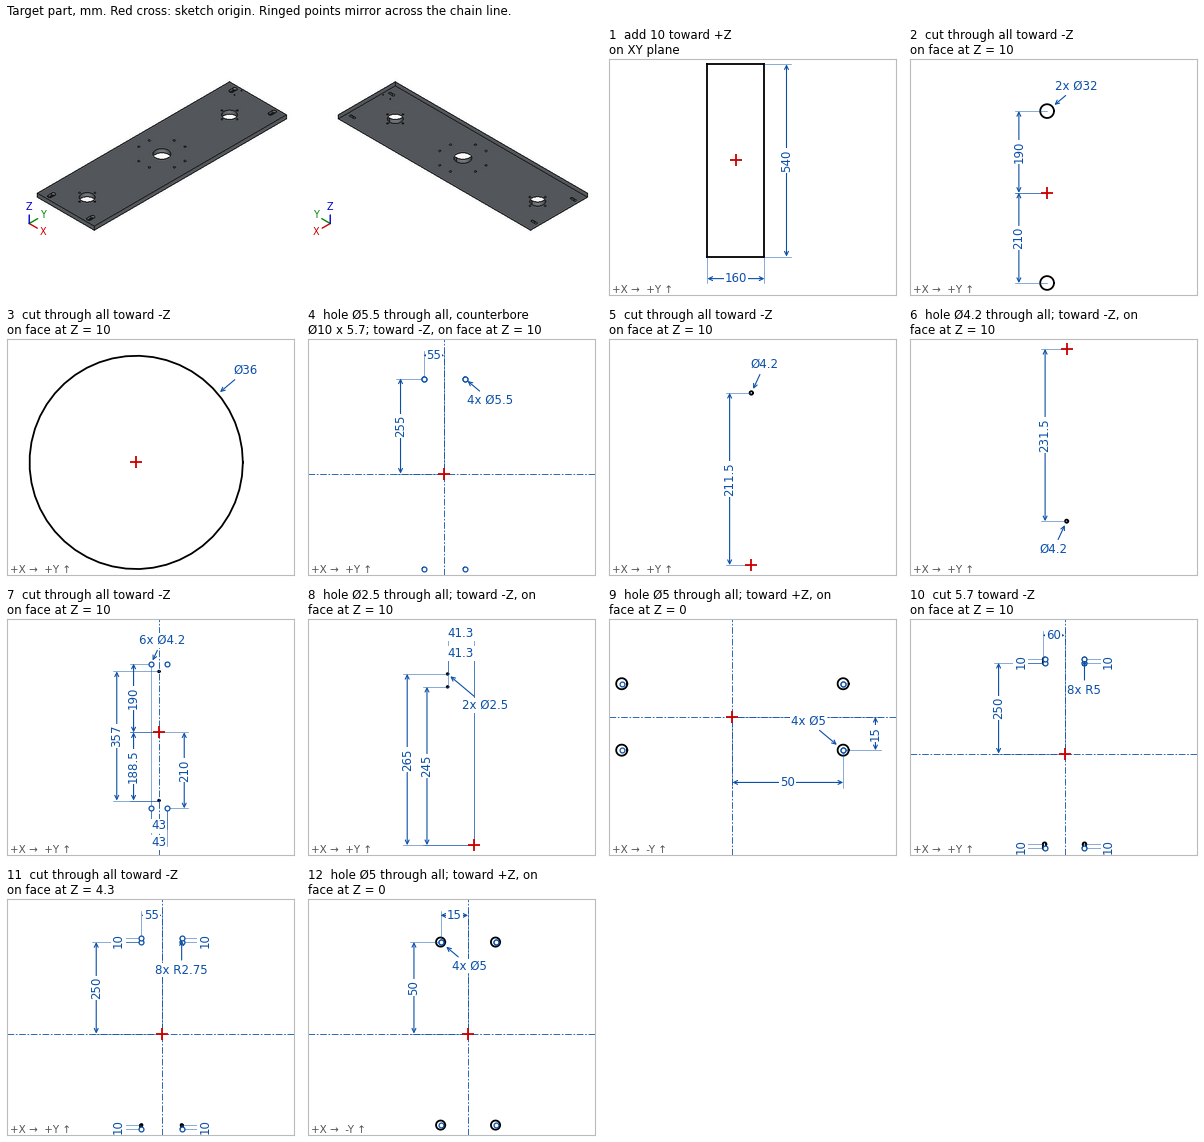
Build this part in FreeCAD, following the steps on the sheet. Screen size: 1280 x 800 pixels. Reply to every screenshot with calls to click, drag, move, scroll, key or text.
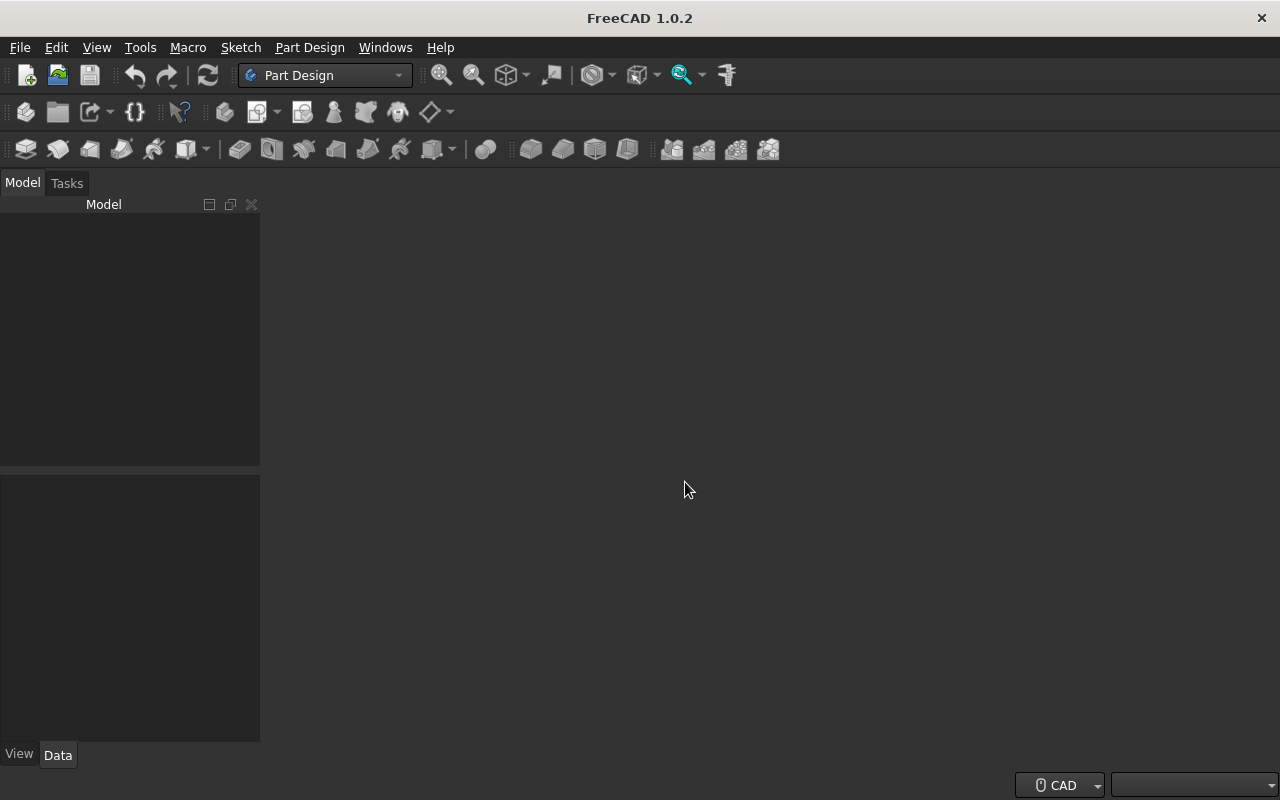
key(ctrl+n)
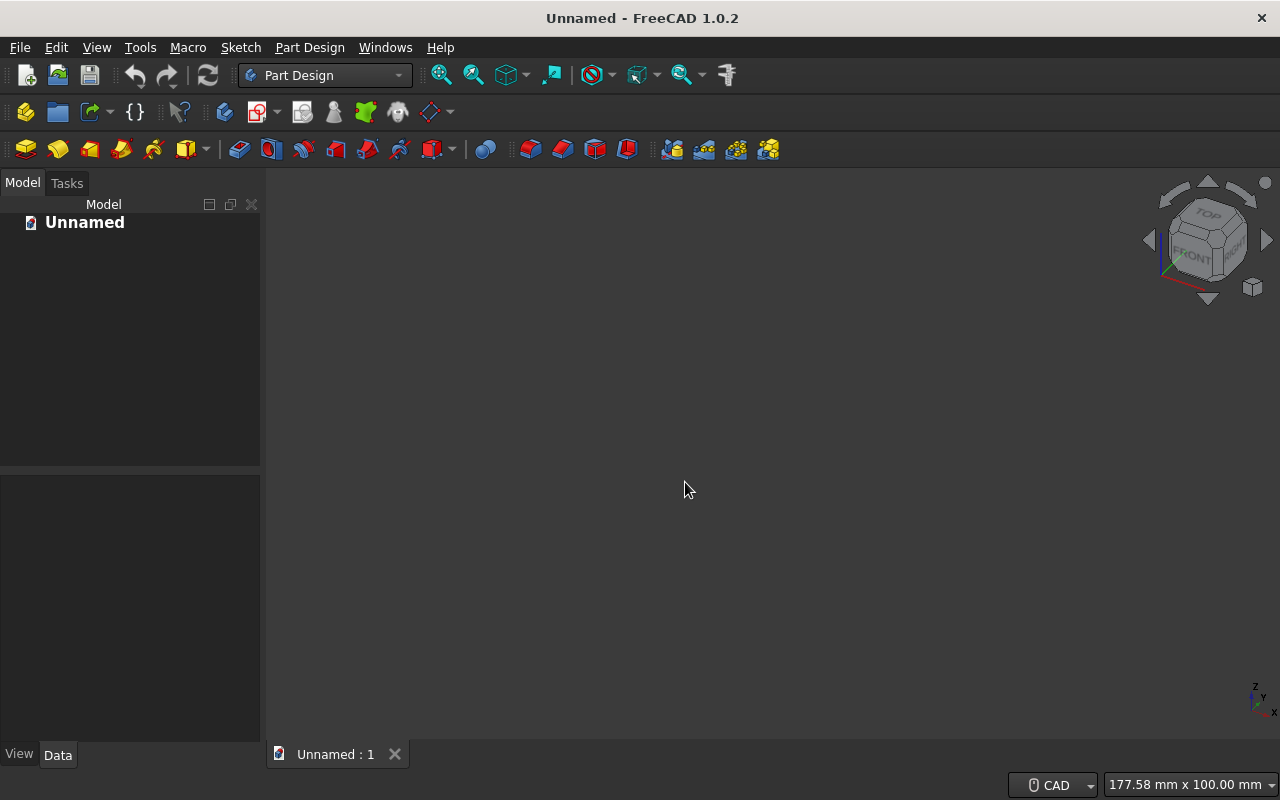
click(258, 112)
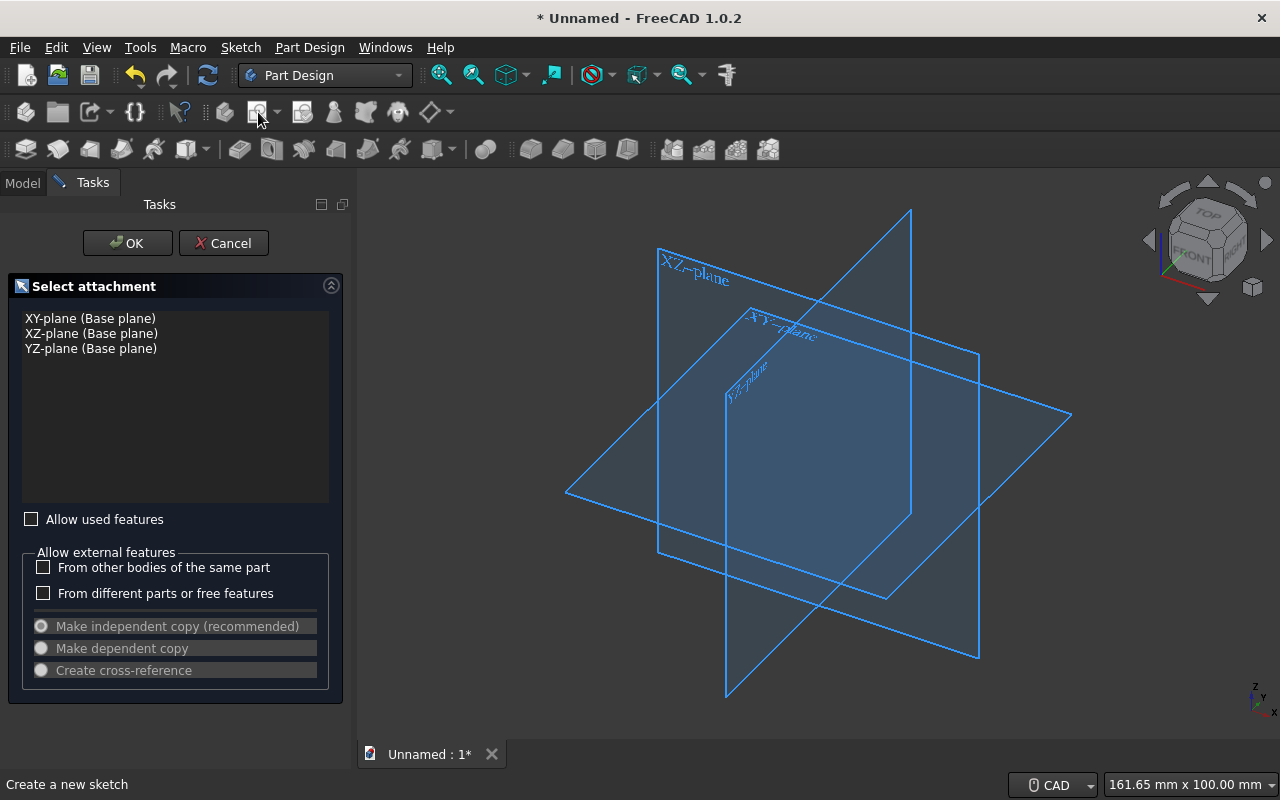
click(82, 318)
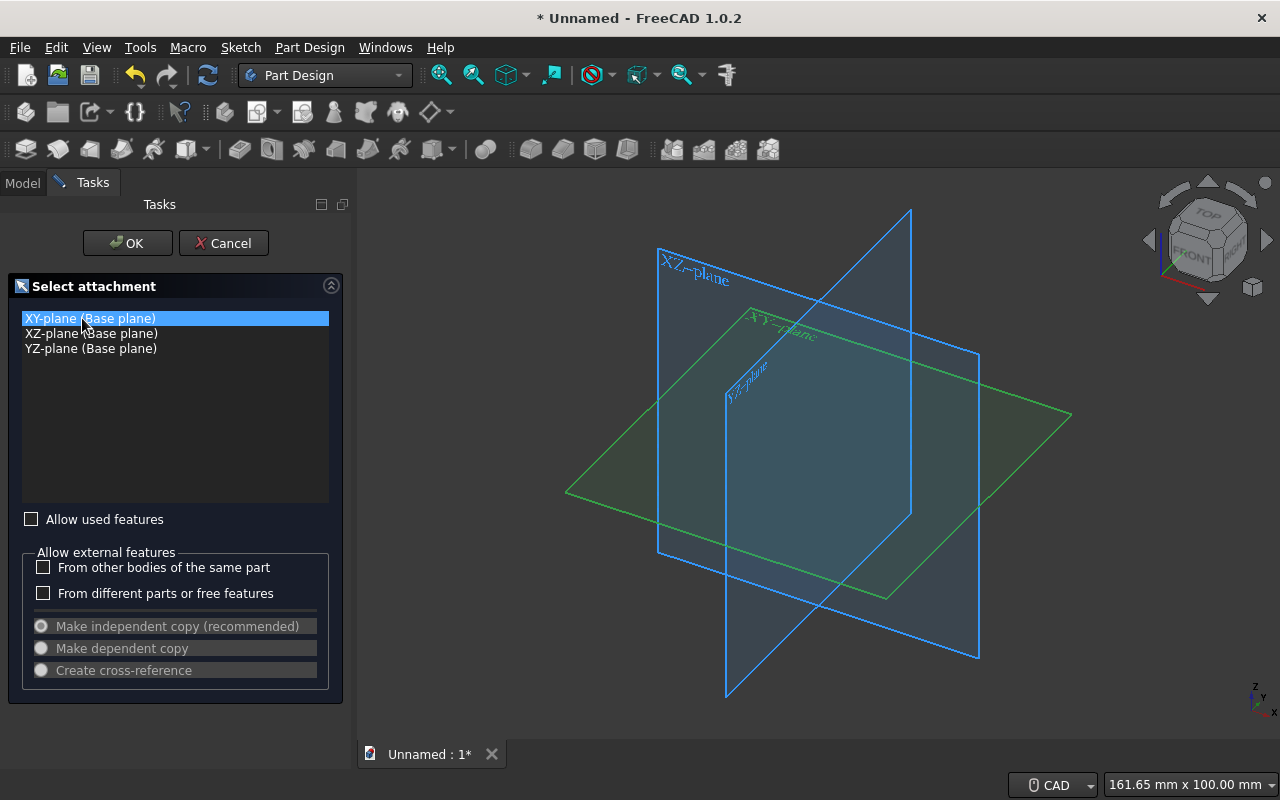
click(128, 243)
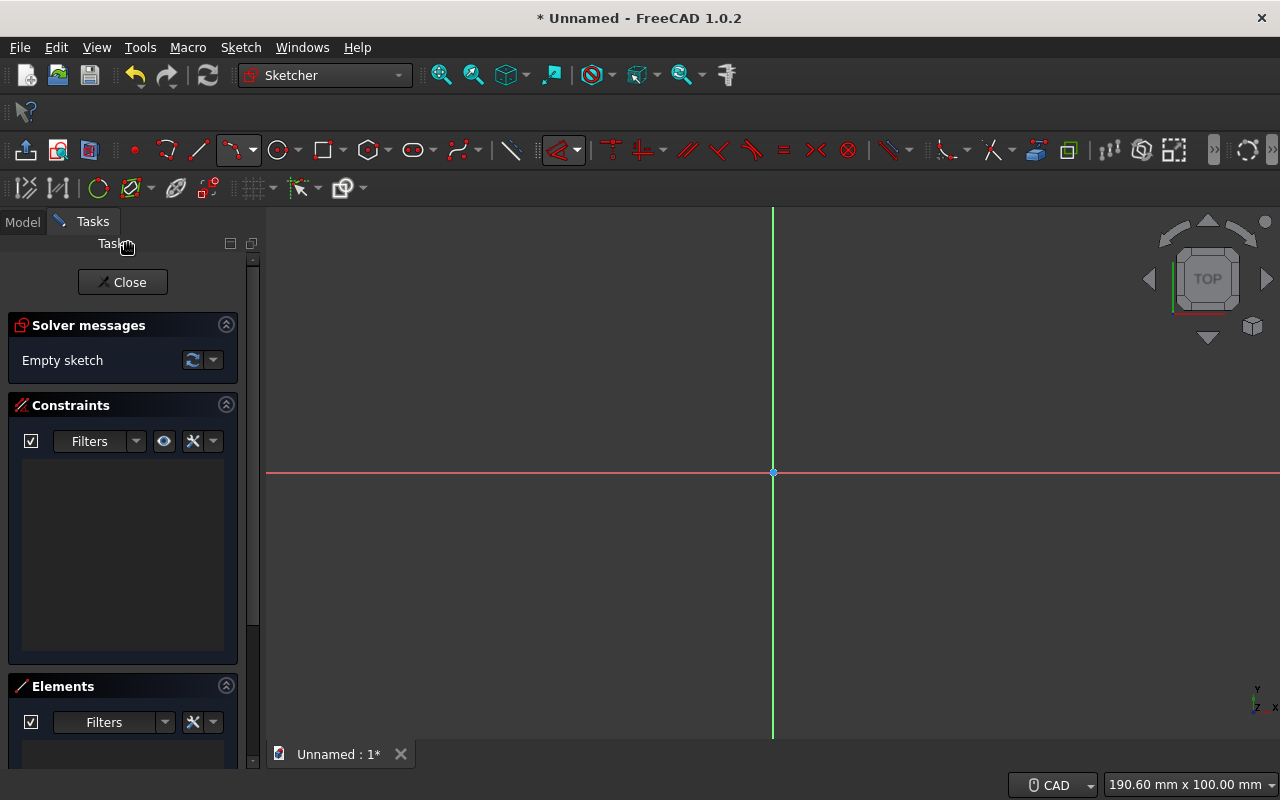
scroll(696, 473, down, 11)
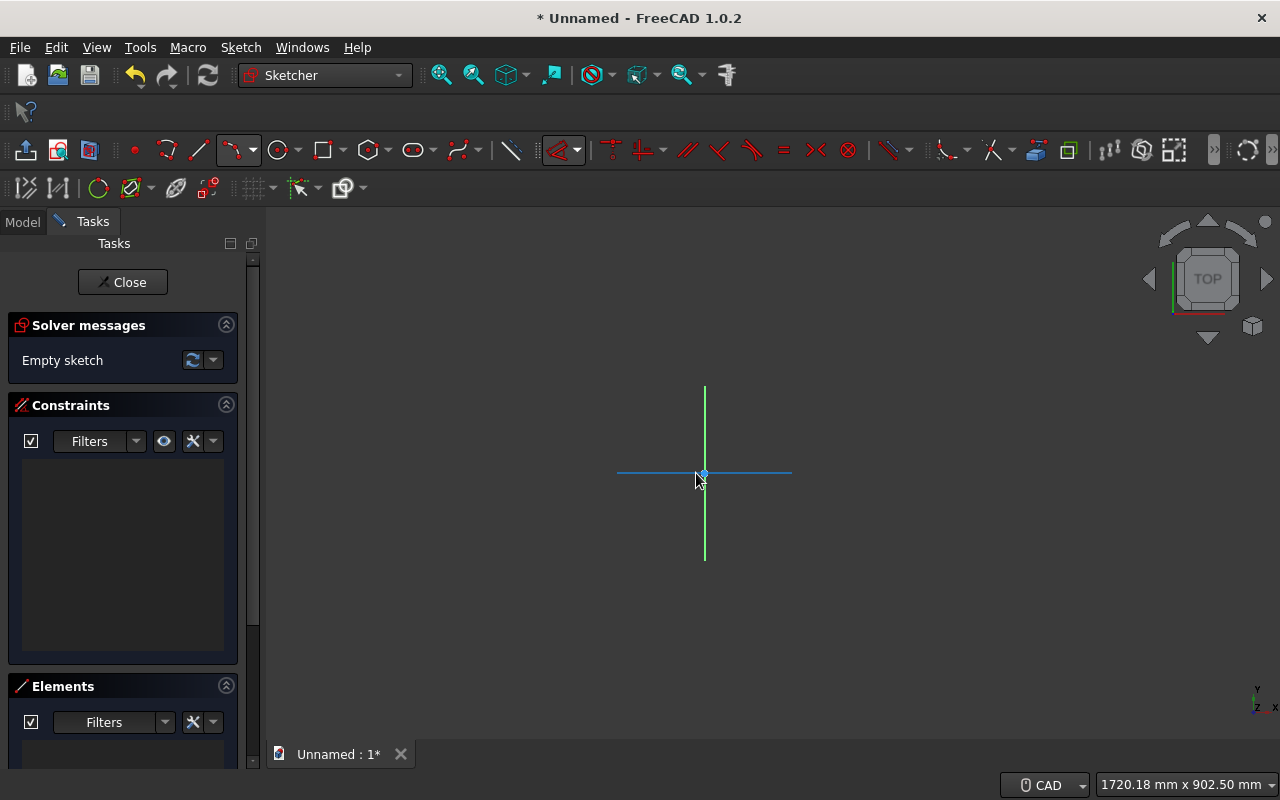
key(g)
key(v)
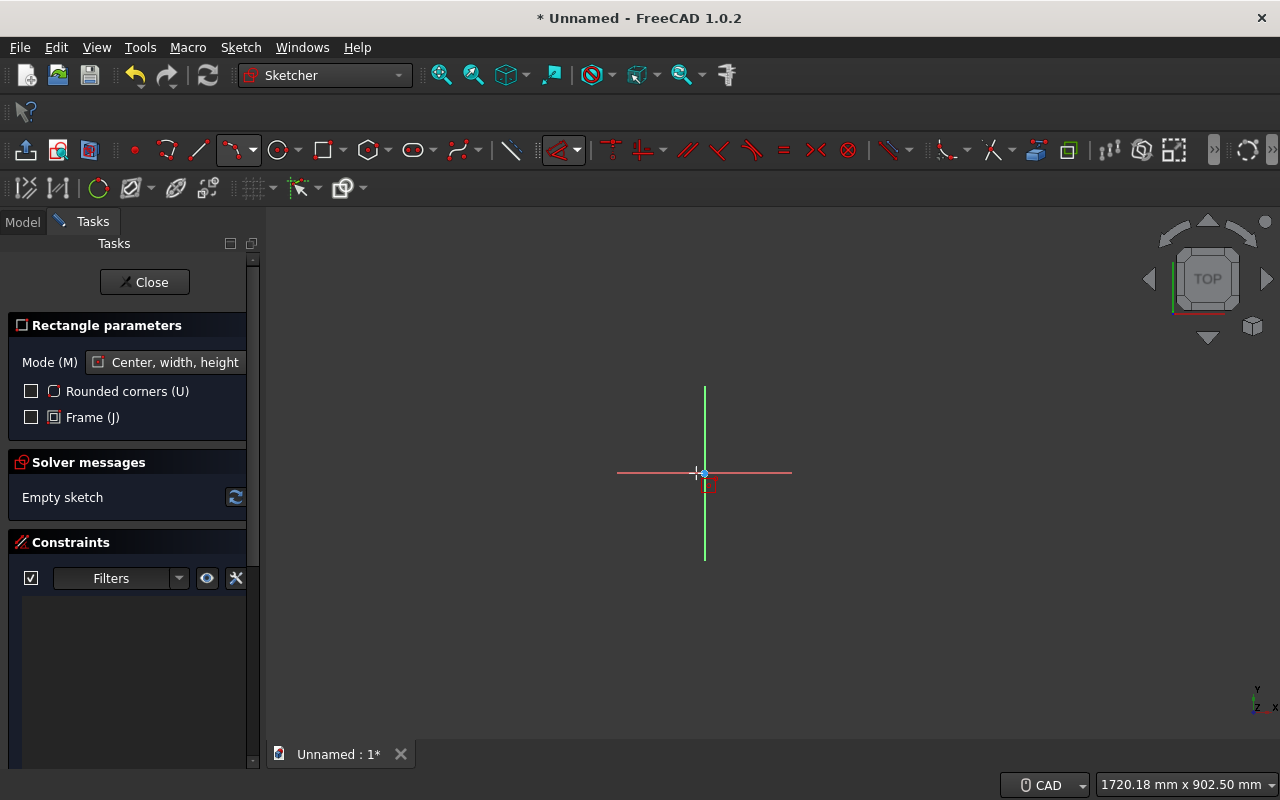
click(705, 473)
move(752, 314)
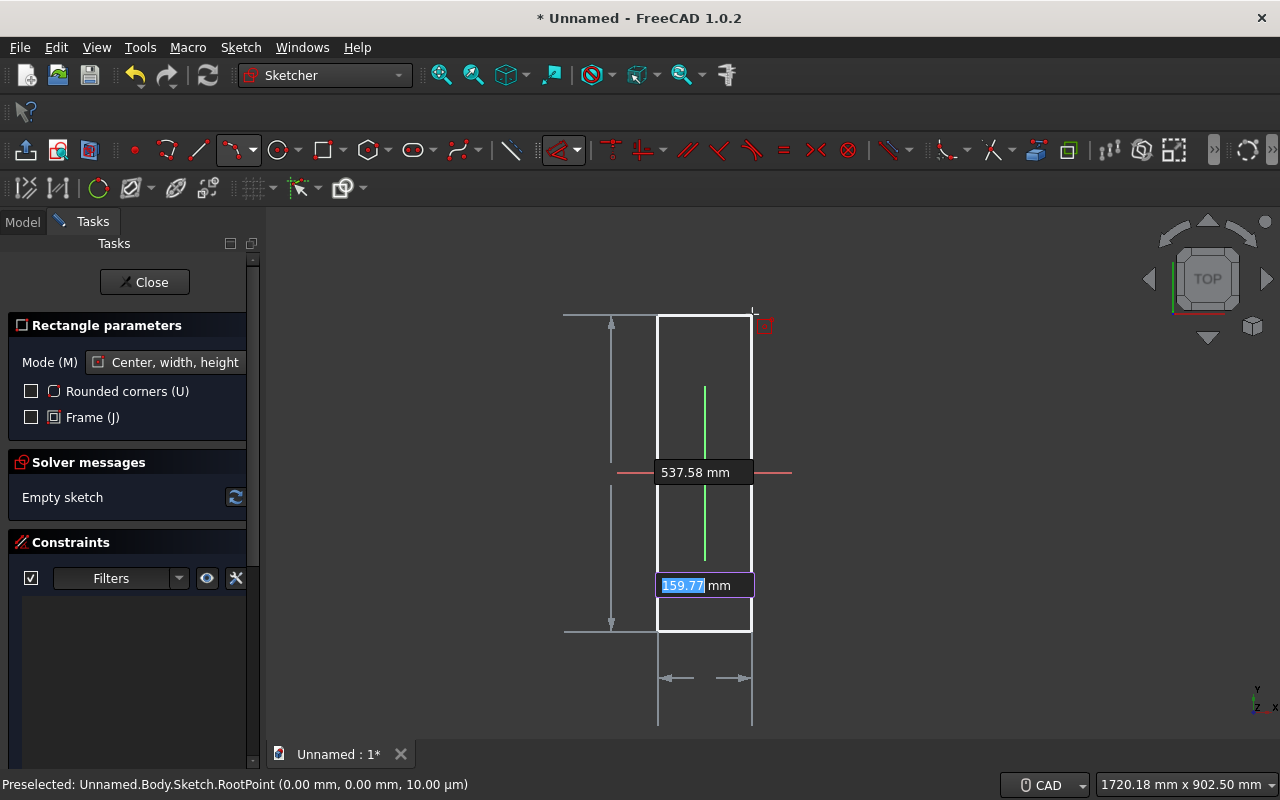
text(160)
key(Tab)
text(540)
key(Return)
key(Escape)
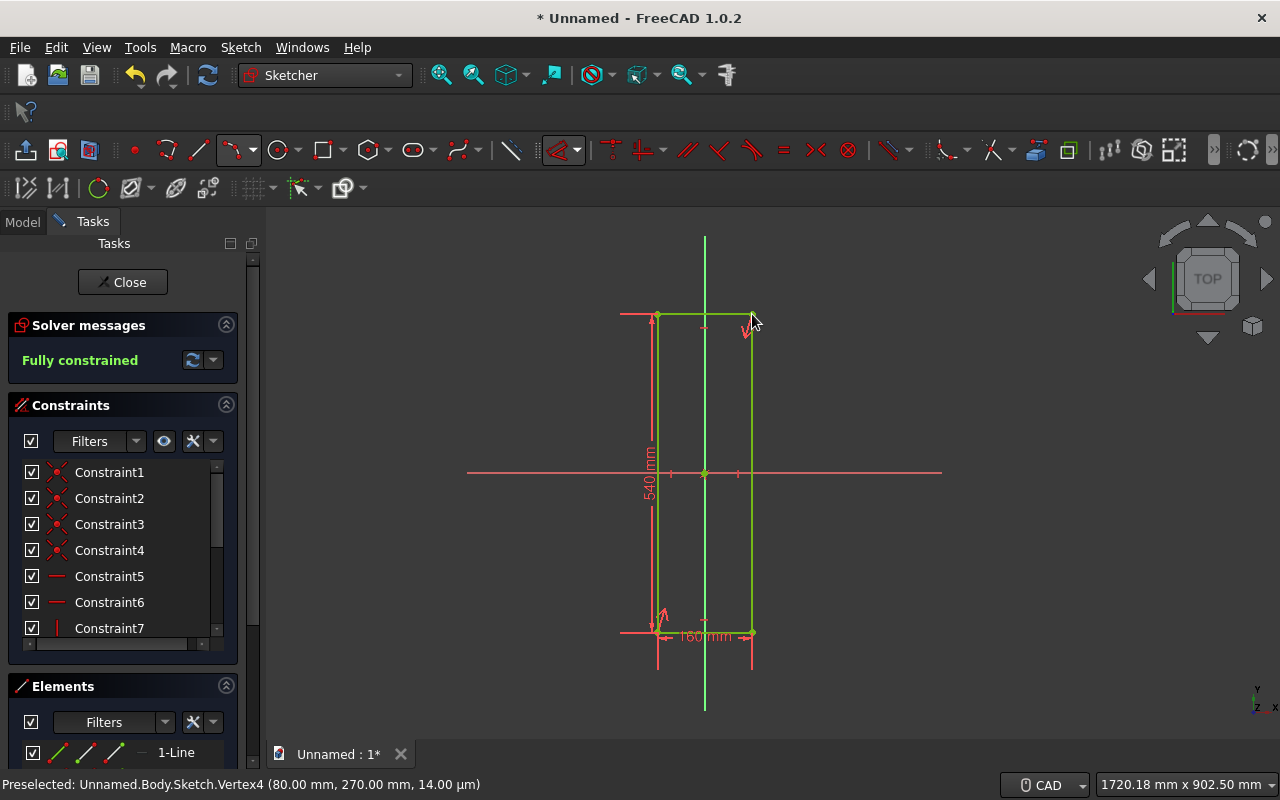
click(123, 282)